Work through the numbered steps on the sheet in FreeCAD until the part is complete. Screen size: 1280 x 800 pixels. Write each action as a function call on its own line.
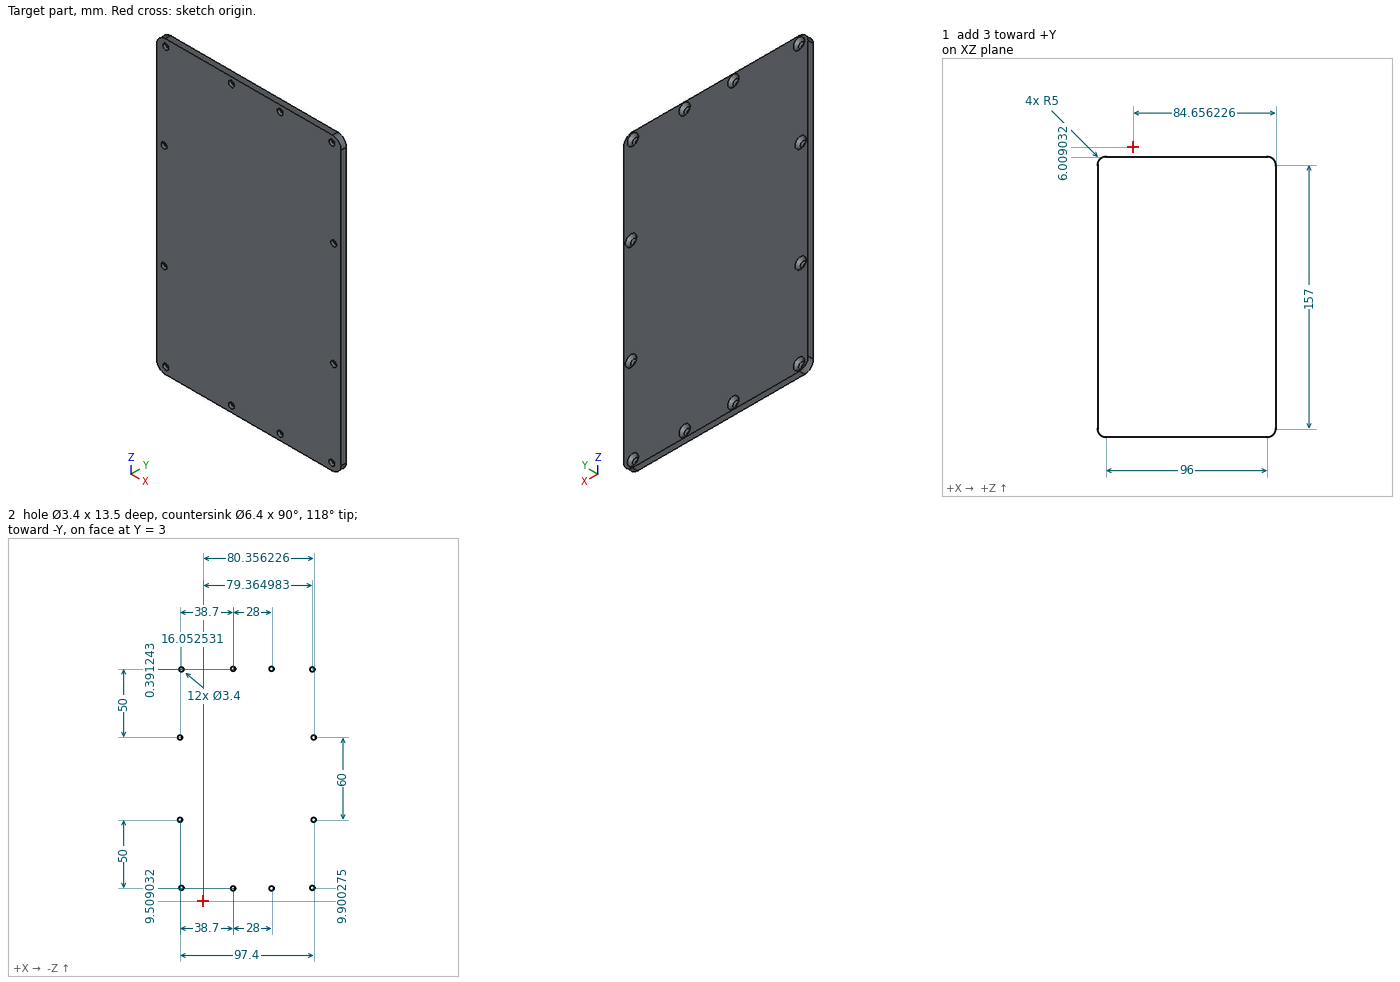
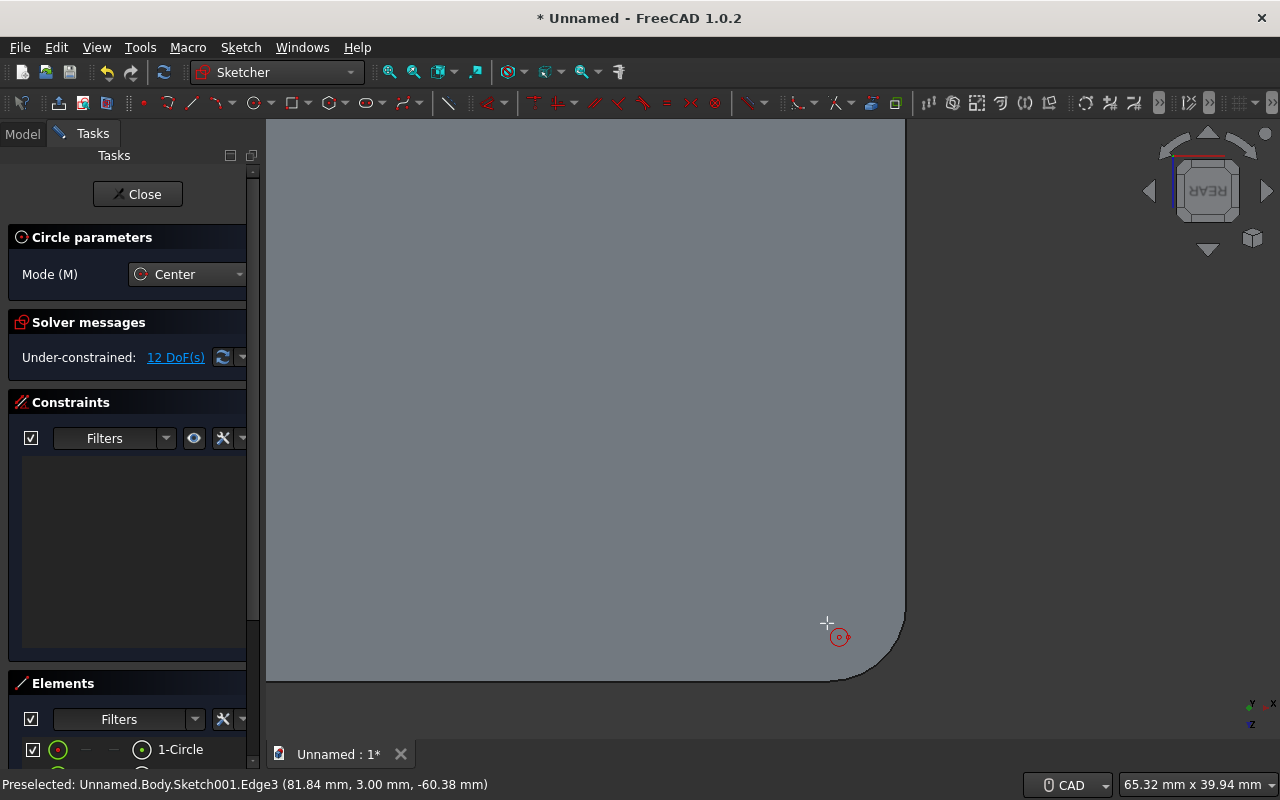
scroll(827, 624, down, 9)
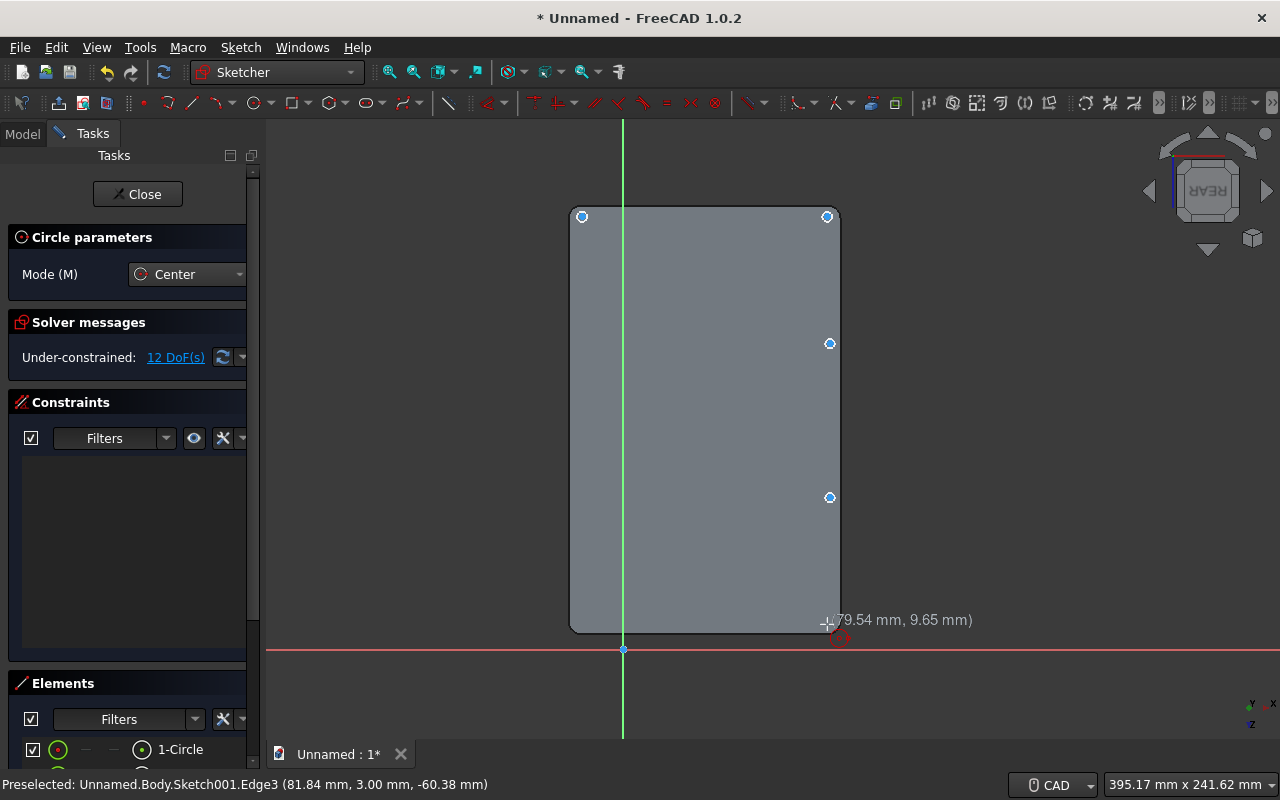
click(827, 624)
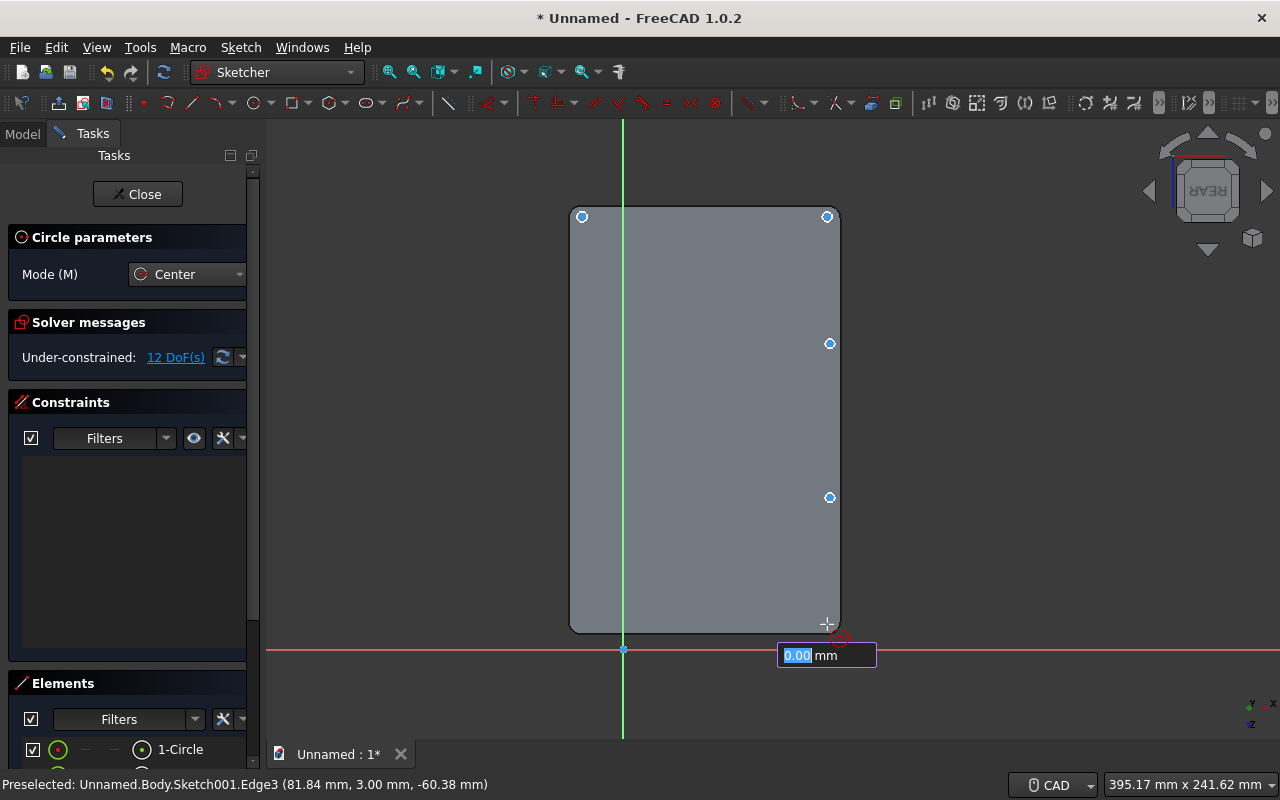
scroll(830, 621, up, 7)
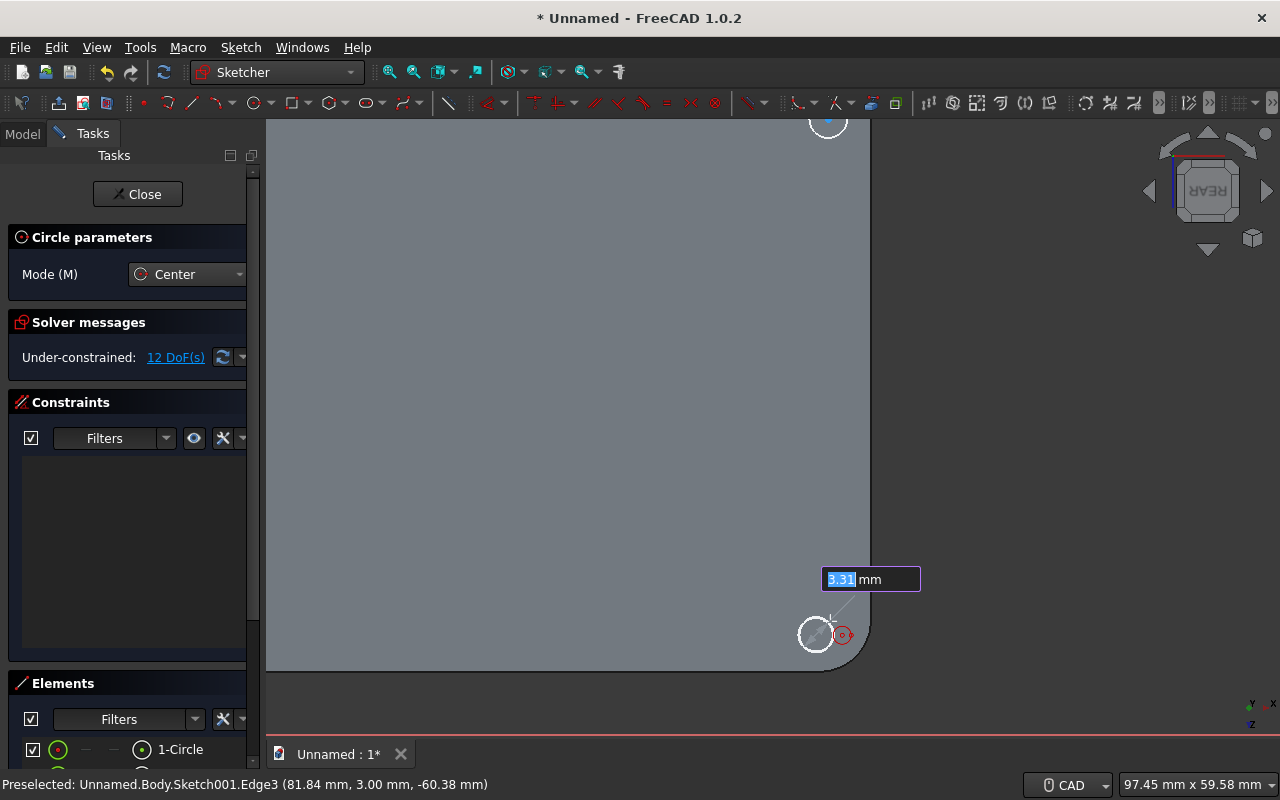
click(829, 619)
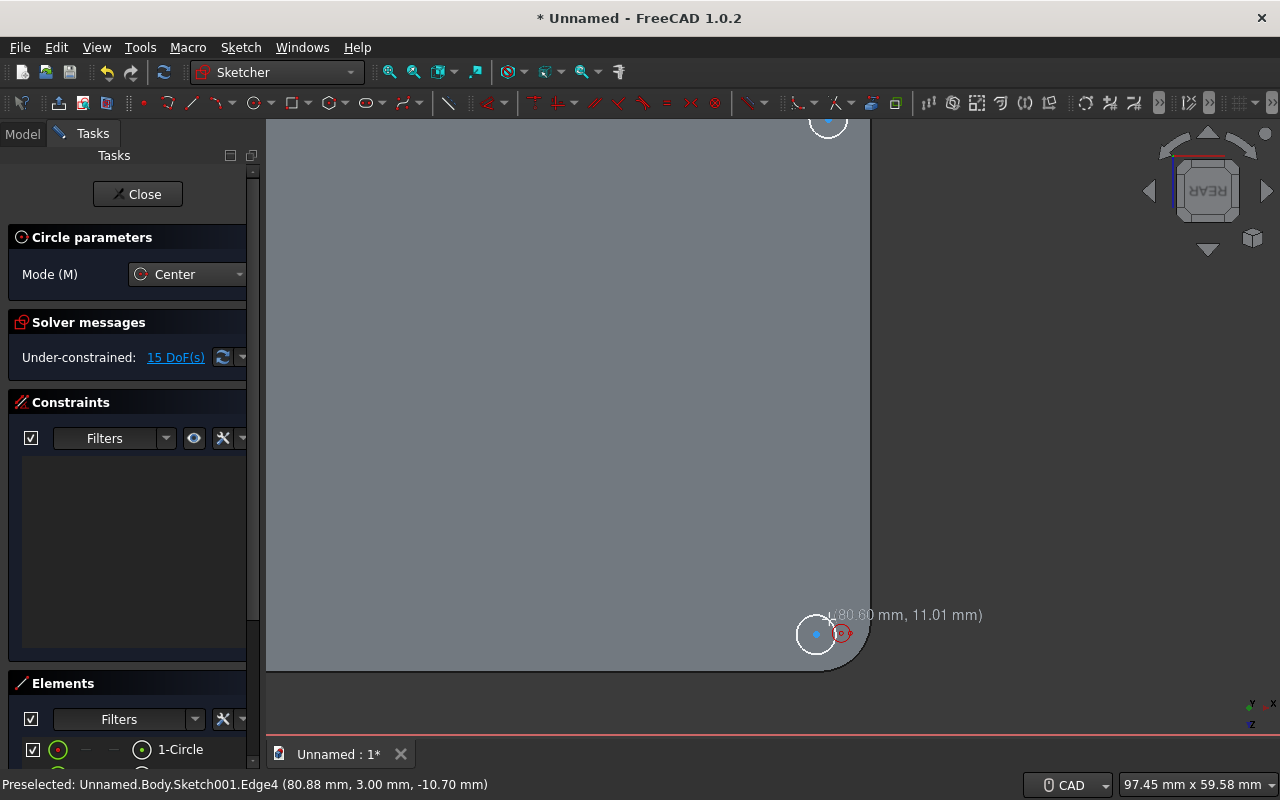
scroll(830, 621, down, 7)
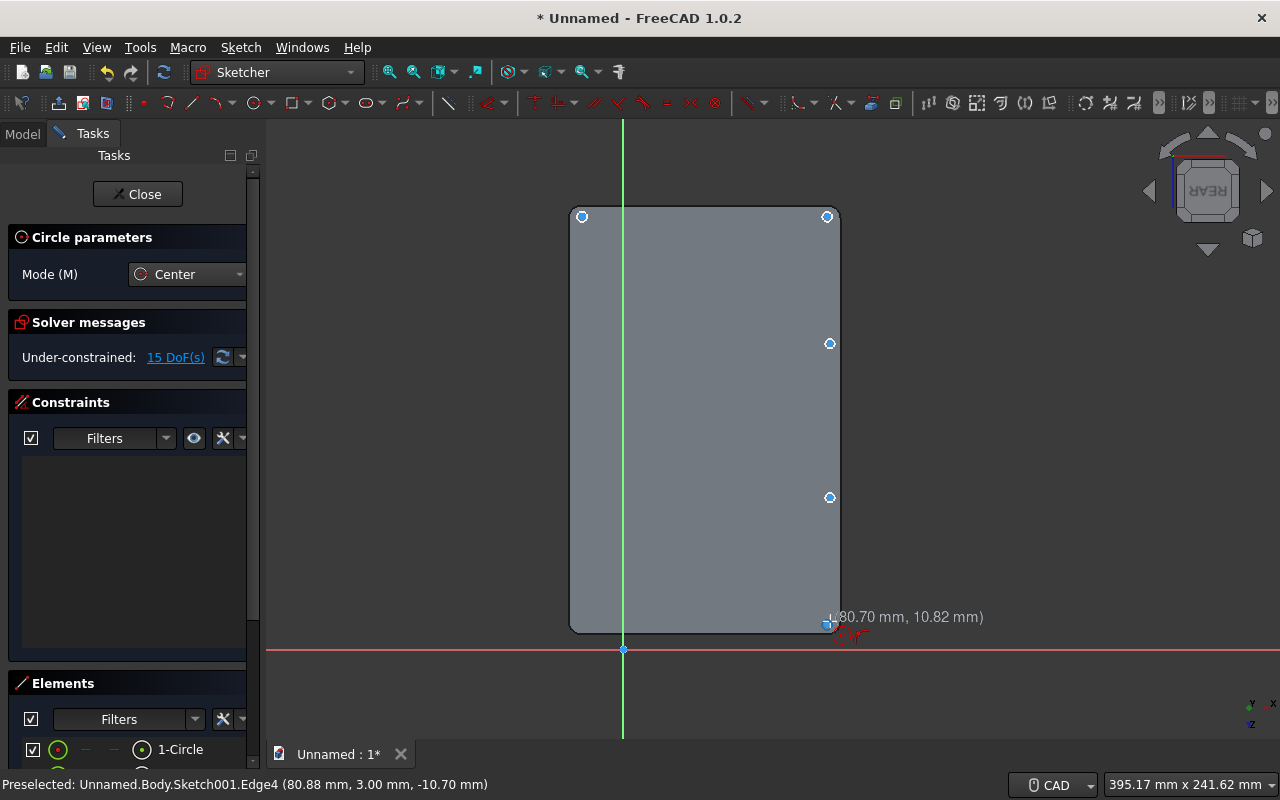
scroll(582, 624, up, 9)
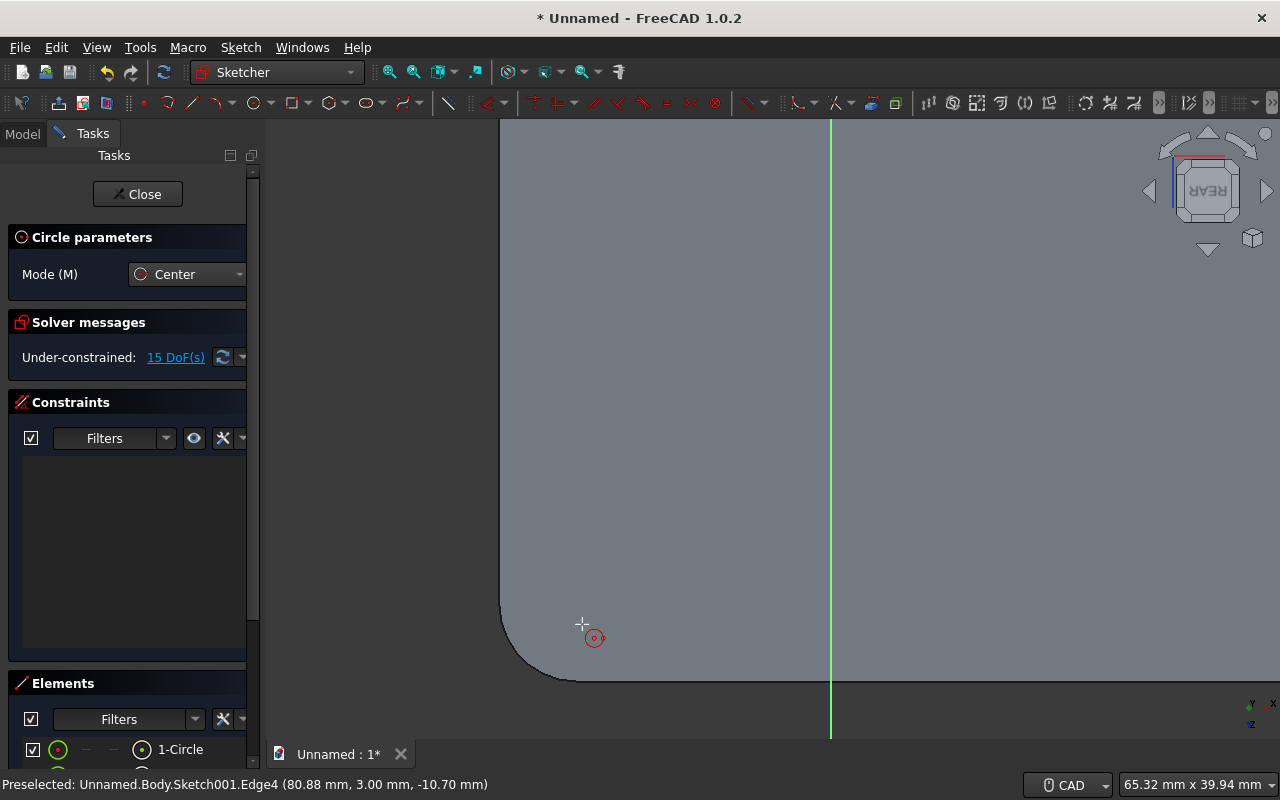
scroll(582, 624, down, 9)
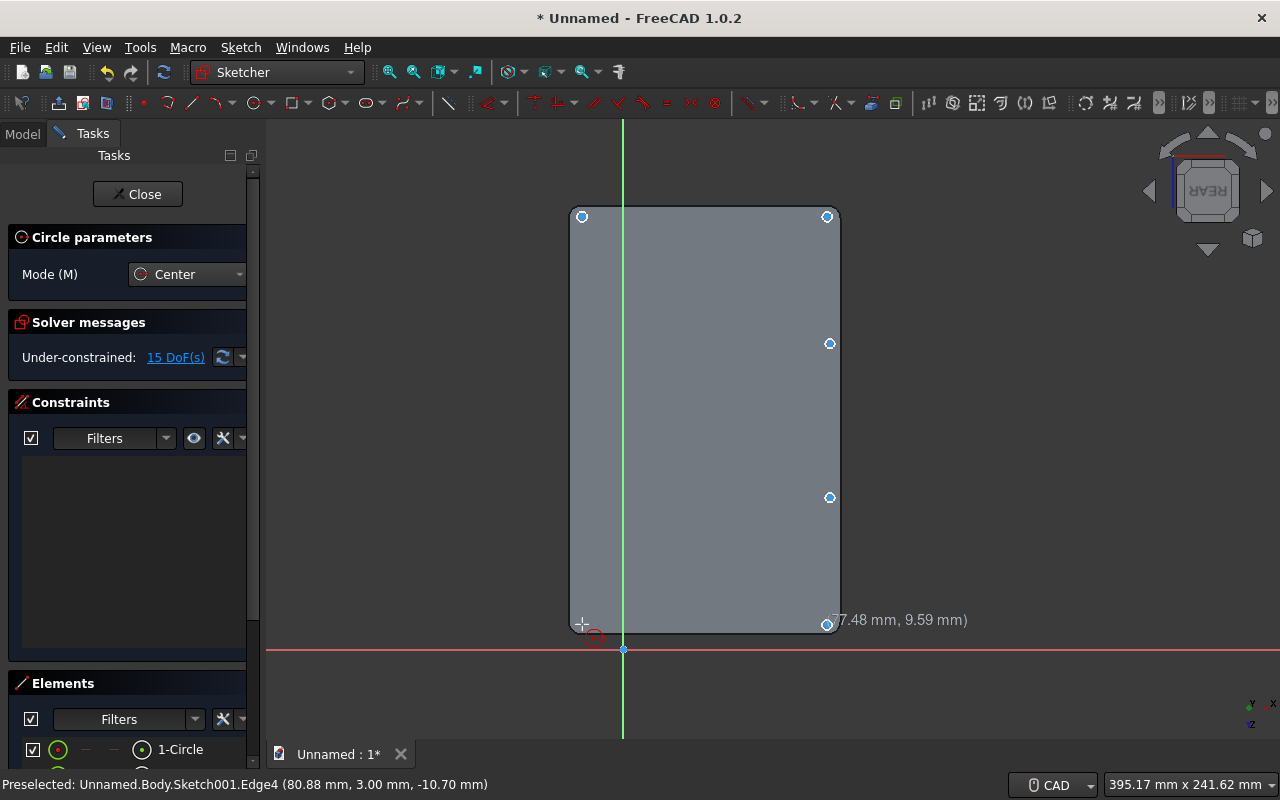
click(582, 624)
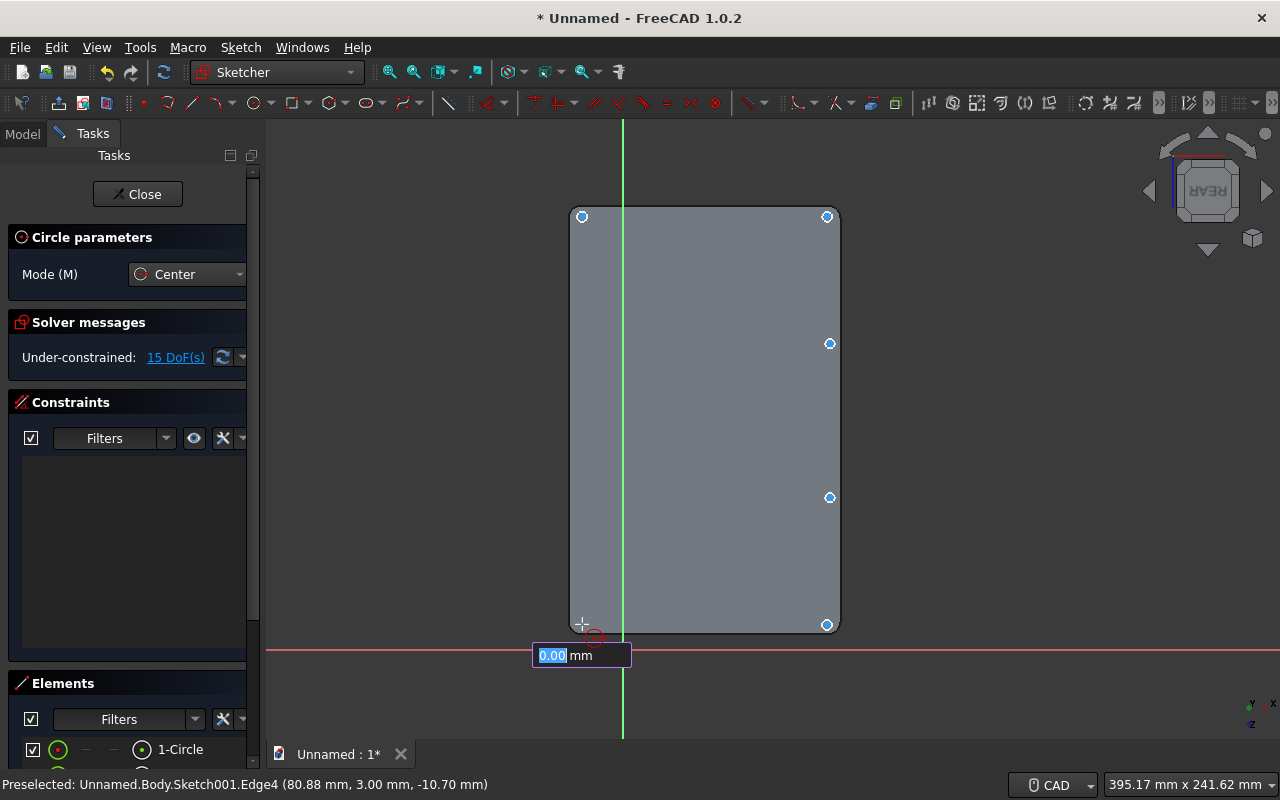
scroll(585, 621, up, 7)